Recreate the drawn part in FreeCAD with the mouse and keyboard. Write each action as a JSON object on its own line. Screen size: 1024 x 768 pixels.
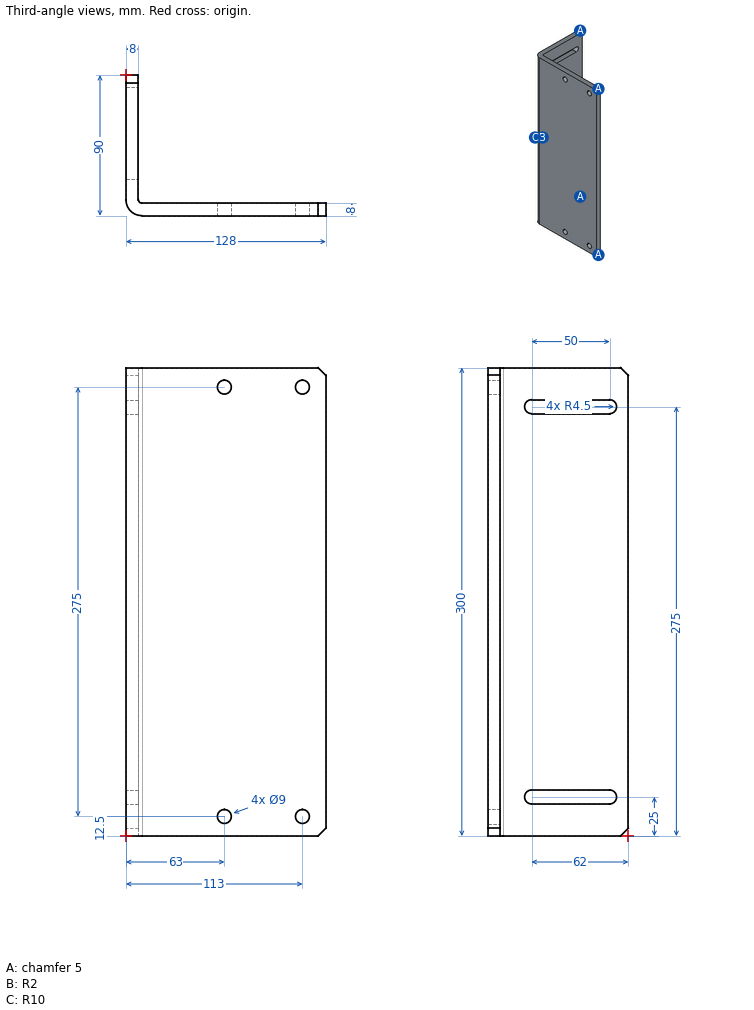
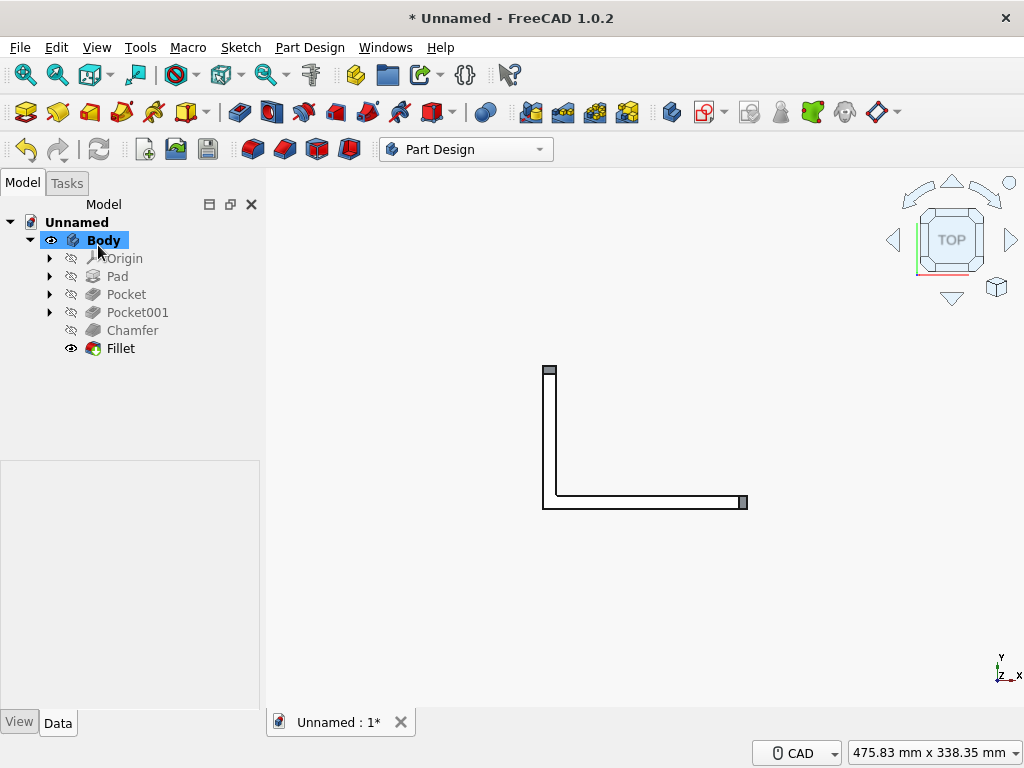
{"action": "key", "text": "0"}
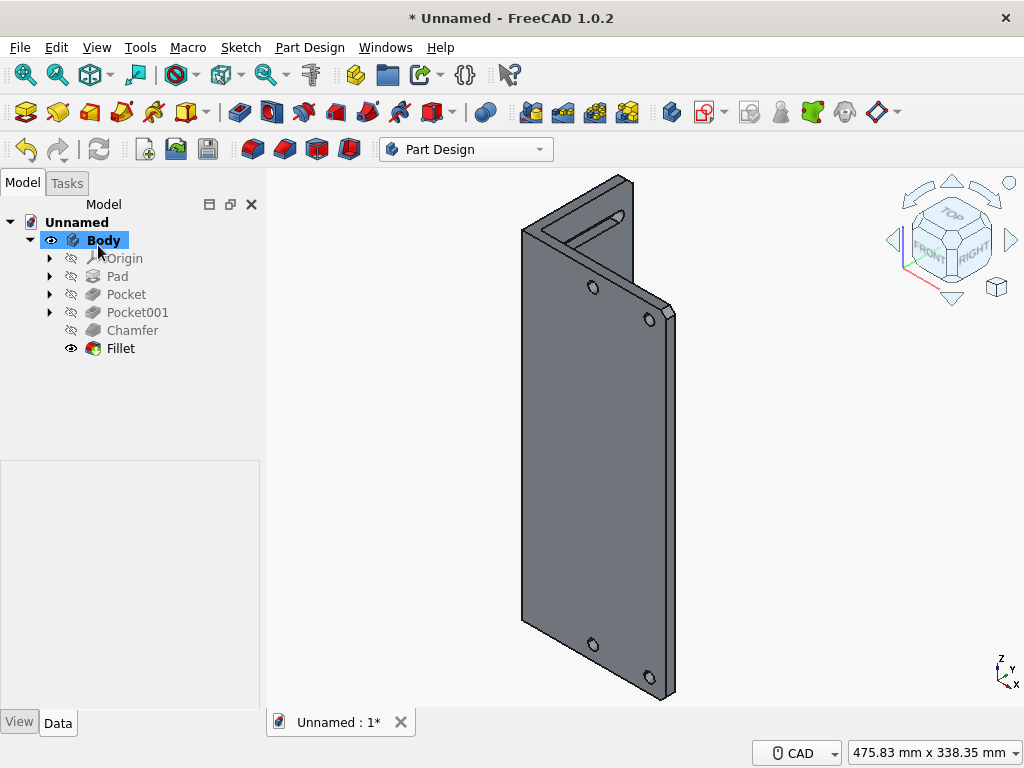
{"action": "key", "text": "1"}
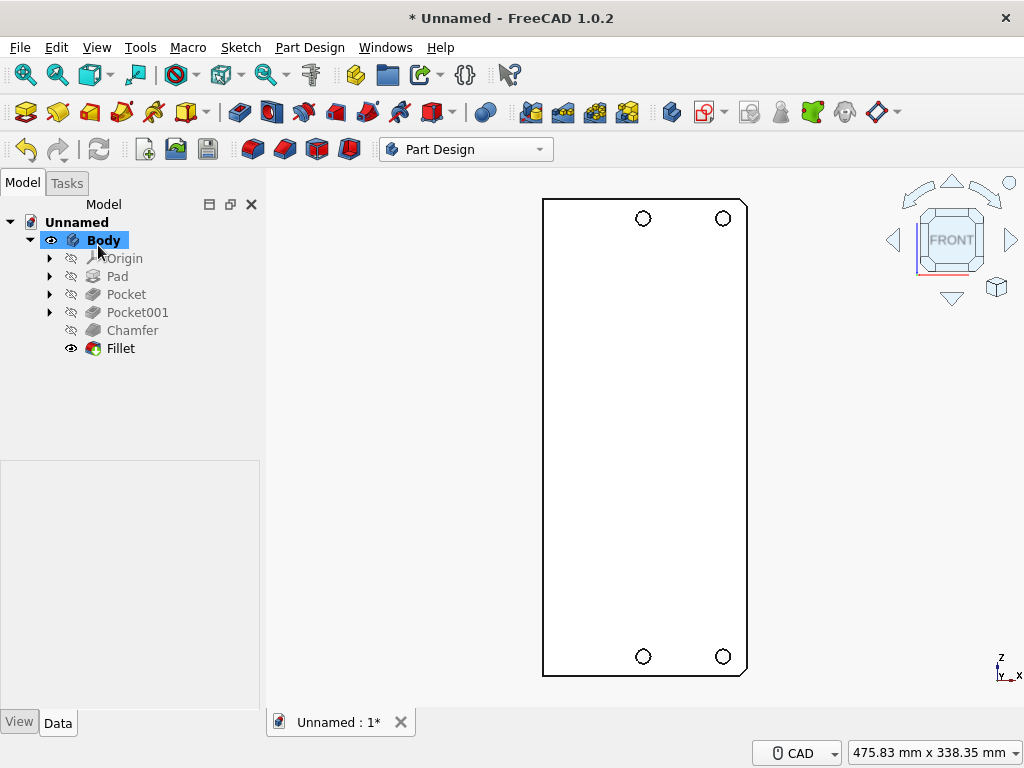
{"action": "left_click", "coordinate": [543, 437]}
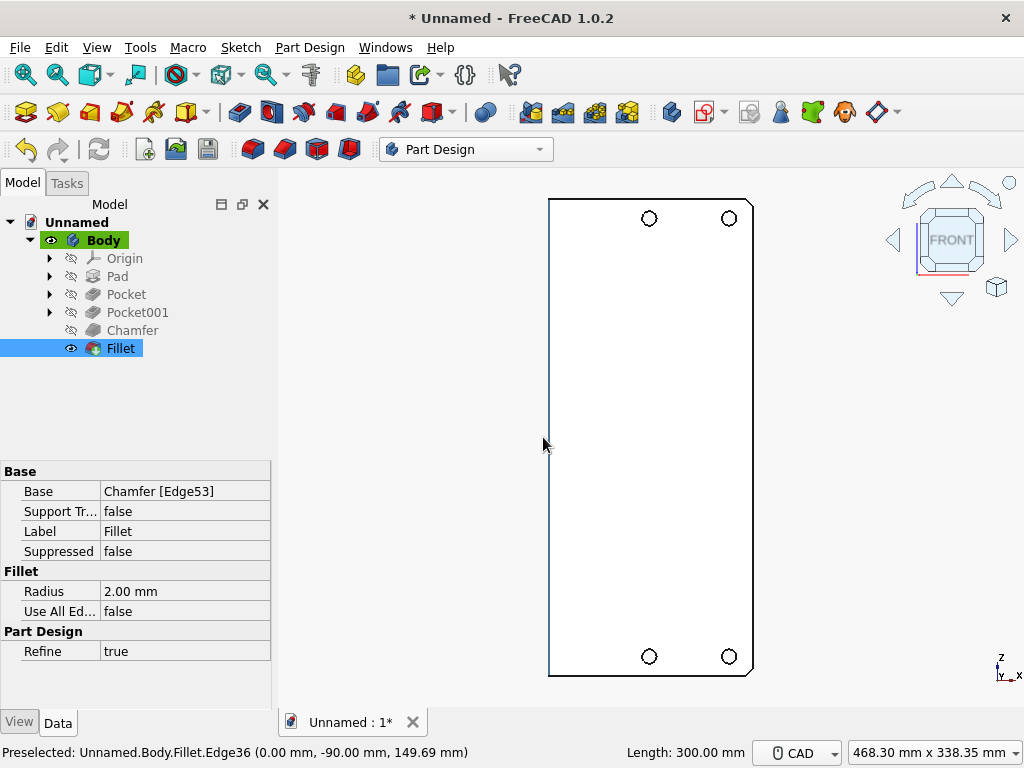
{"action": "left_click", "coordinate": [254, 150]}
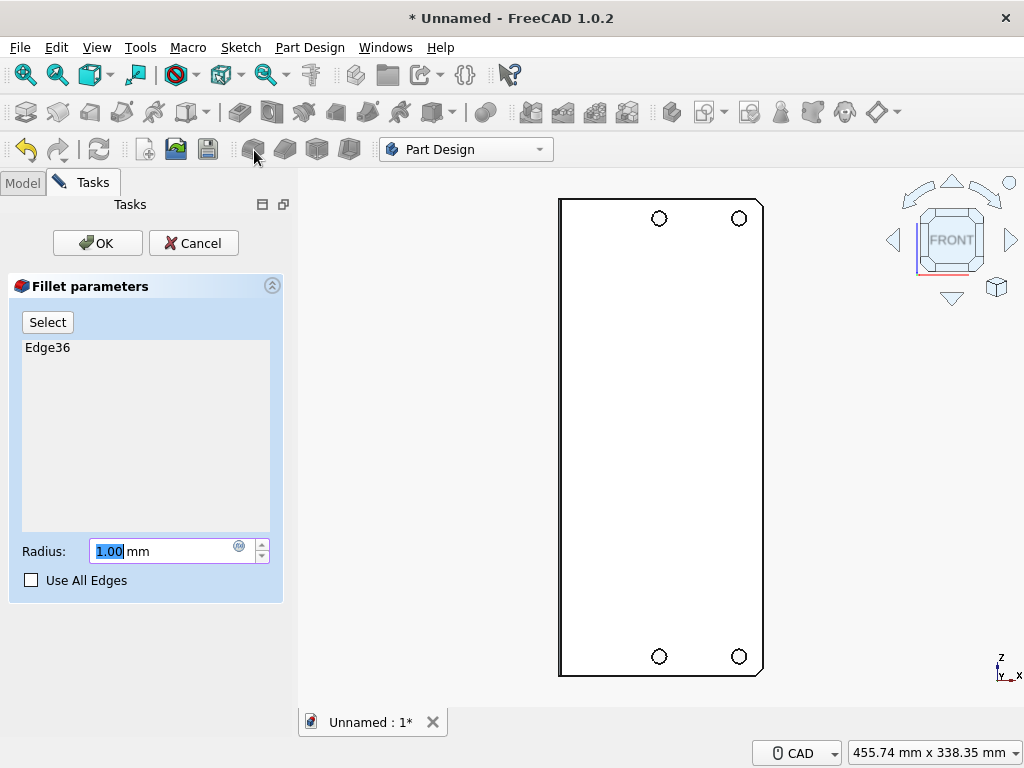
{"action": "type", "text": "10"}
{"action": "key", "text": "Tab"}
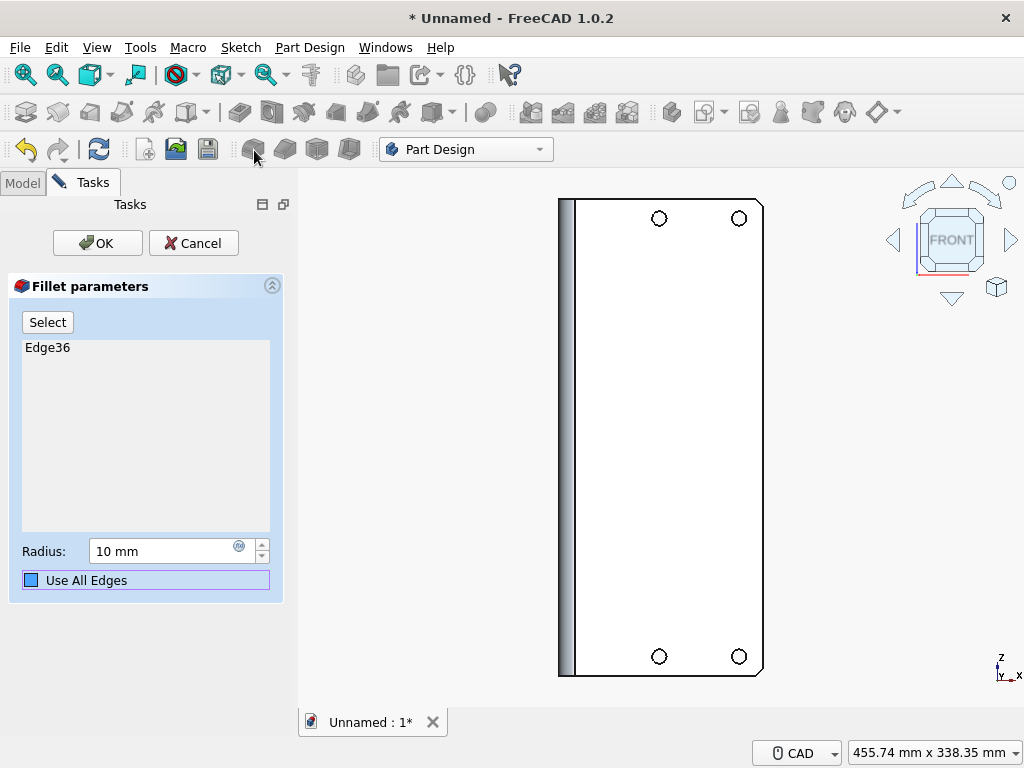
{"action": "left_click", "coordinate": [98, 243]}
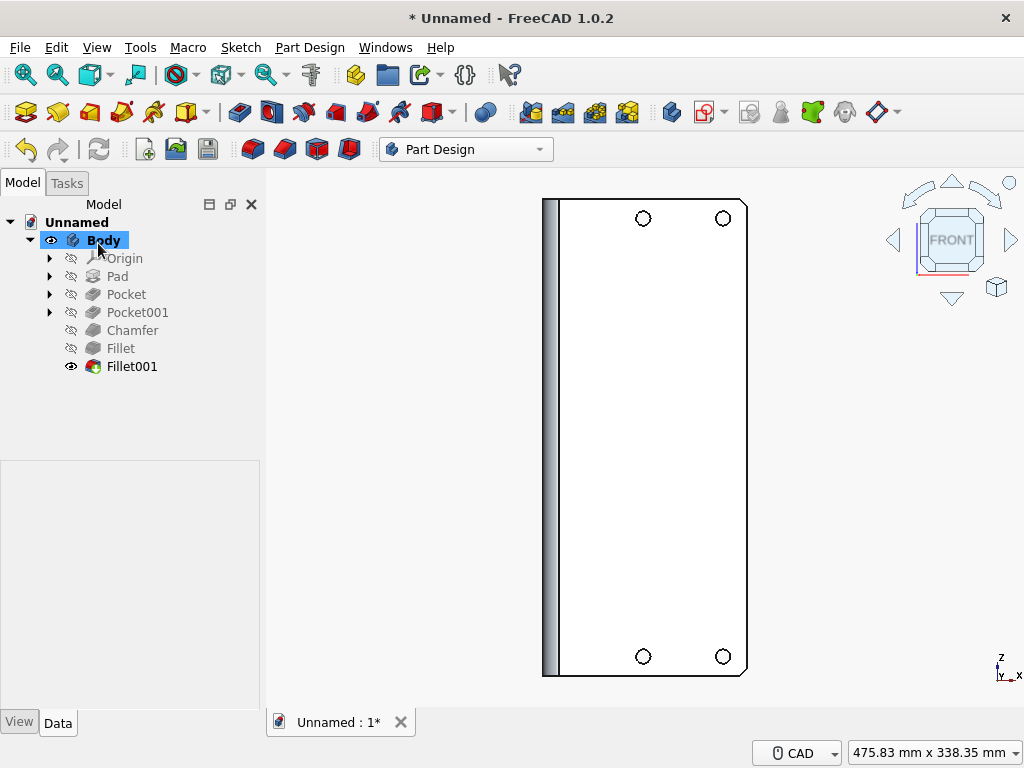
{"action": "key", "text": "0"}